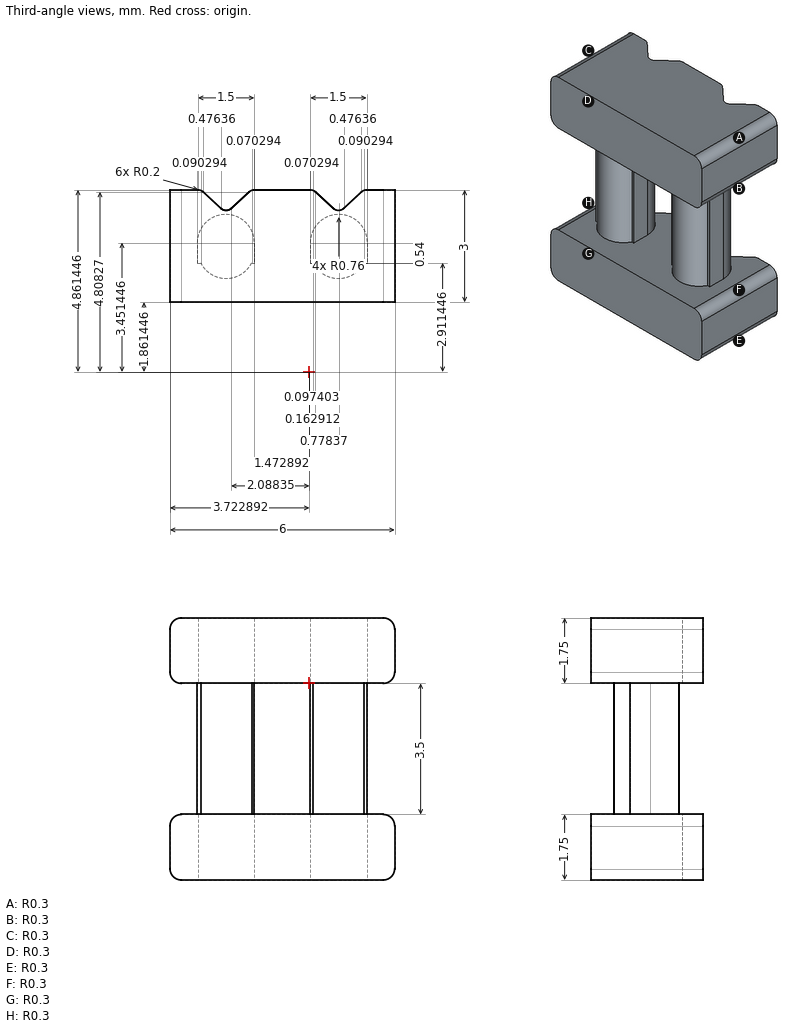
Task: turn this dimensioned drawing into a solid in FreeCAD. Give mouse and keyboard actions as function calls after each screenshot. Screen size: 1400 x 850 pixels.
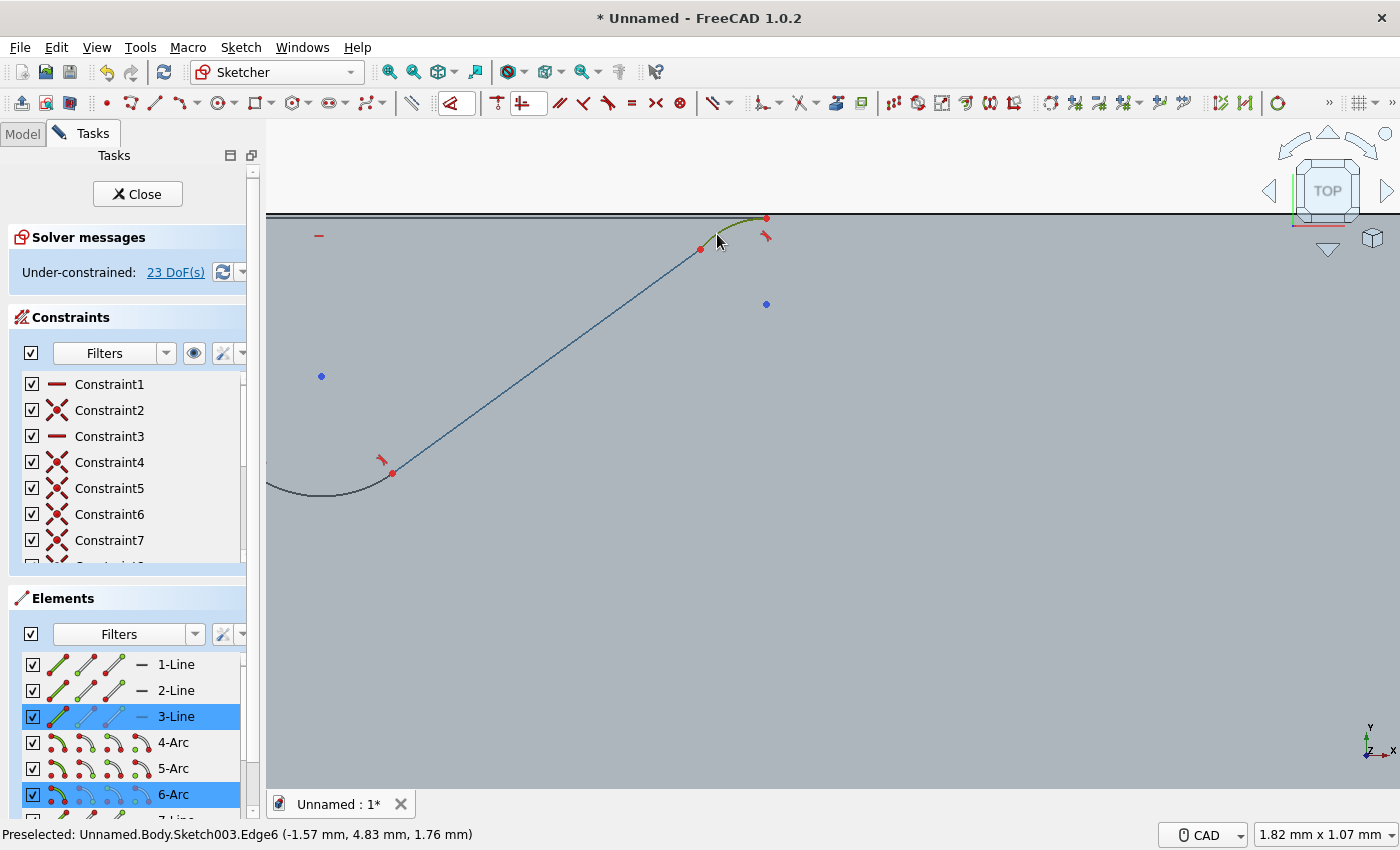
click(608, 104)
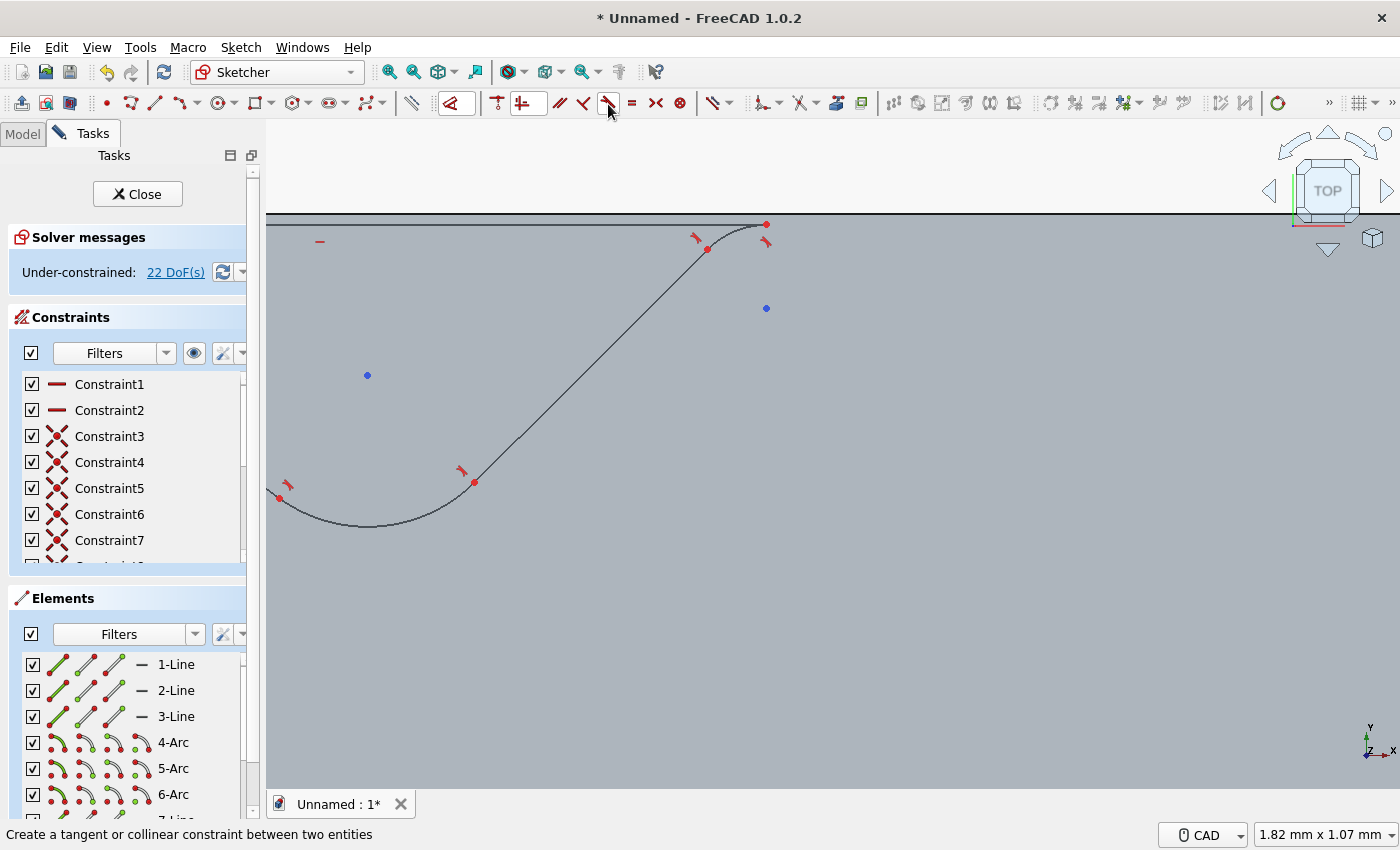
scroll(689, 254, down, 10)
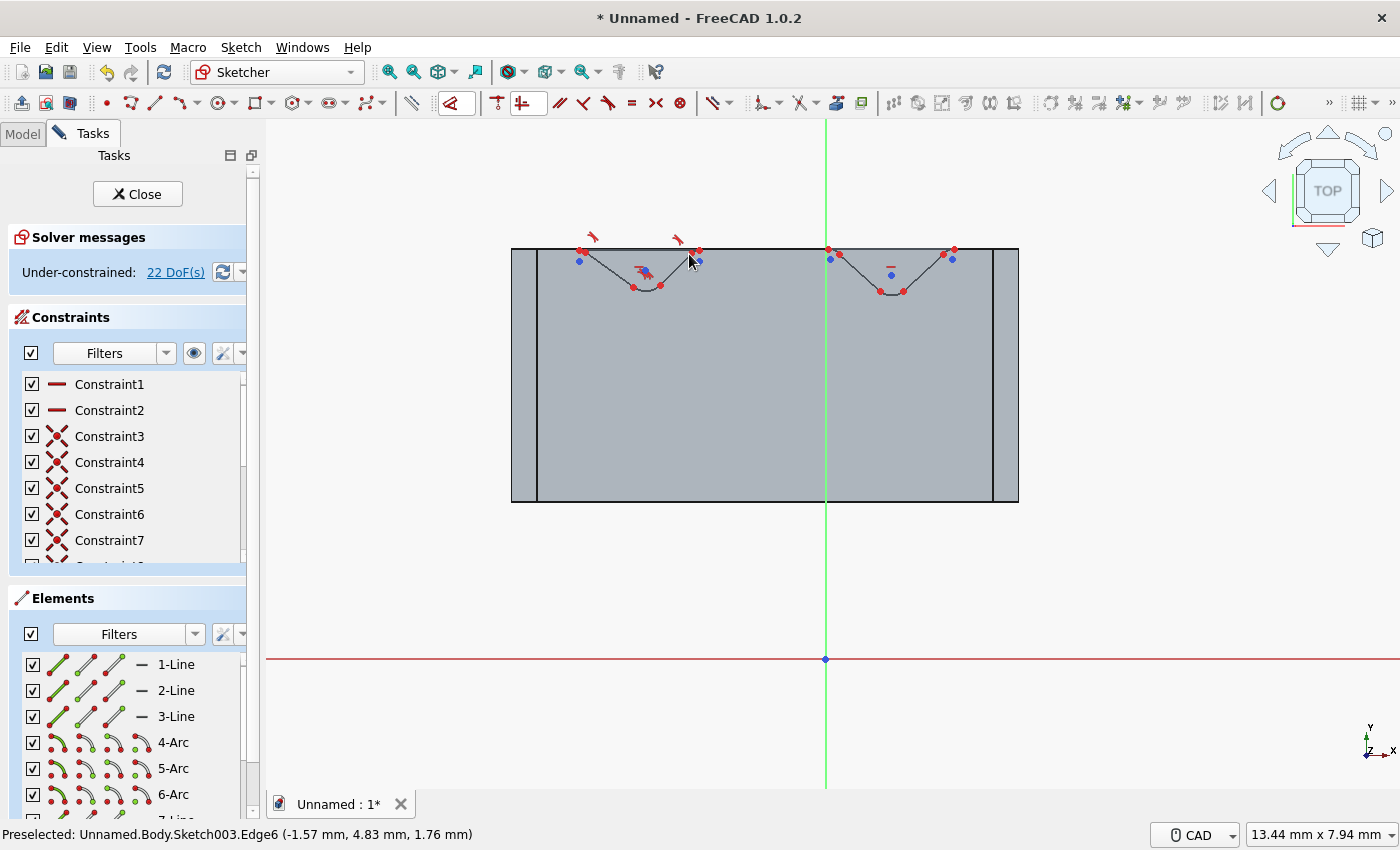
click(852, 266)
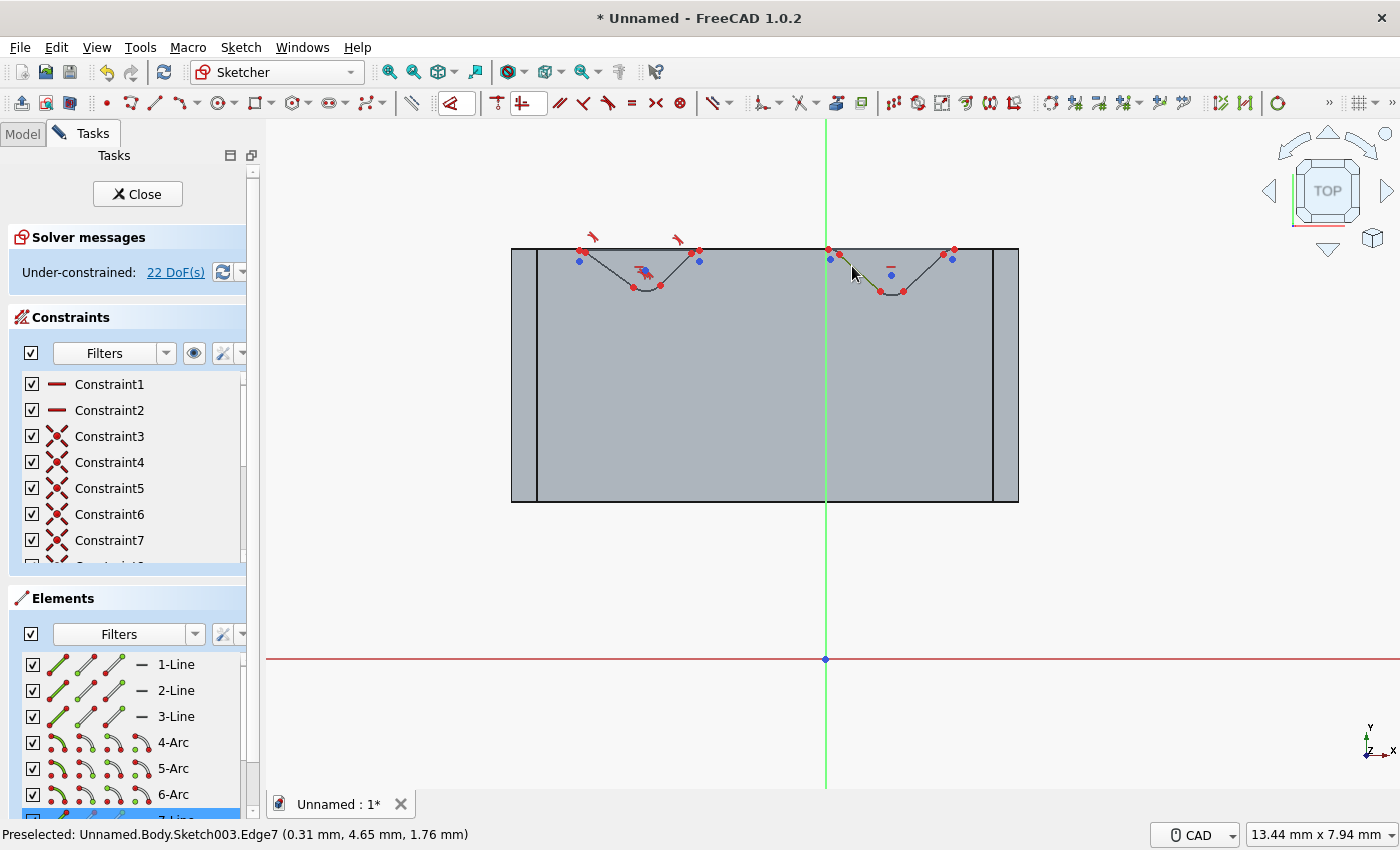
click(892, 295)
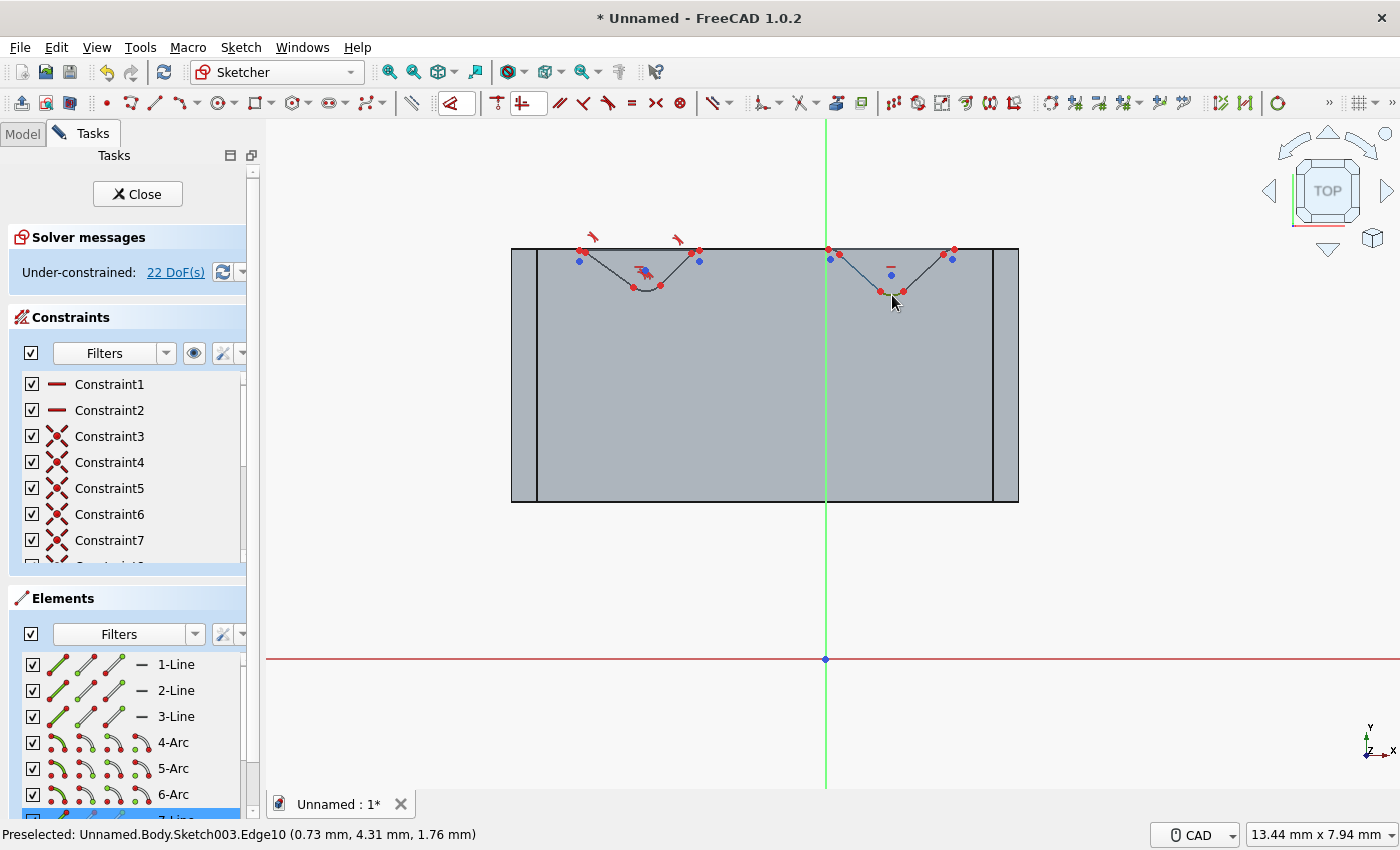
click(608, 104)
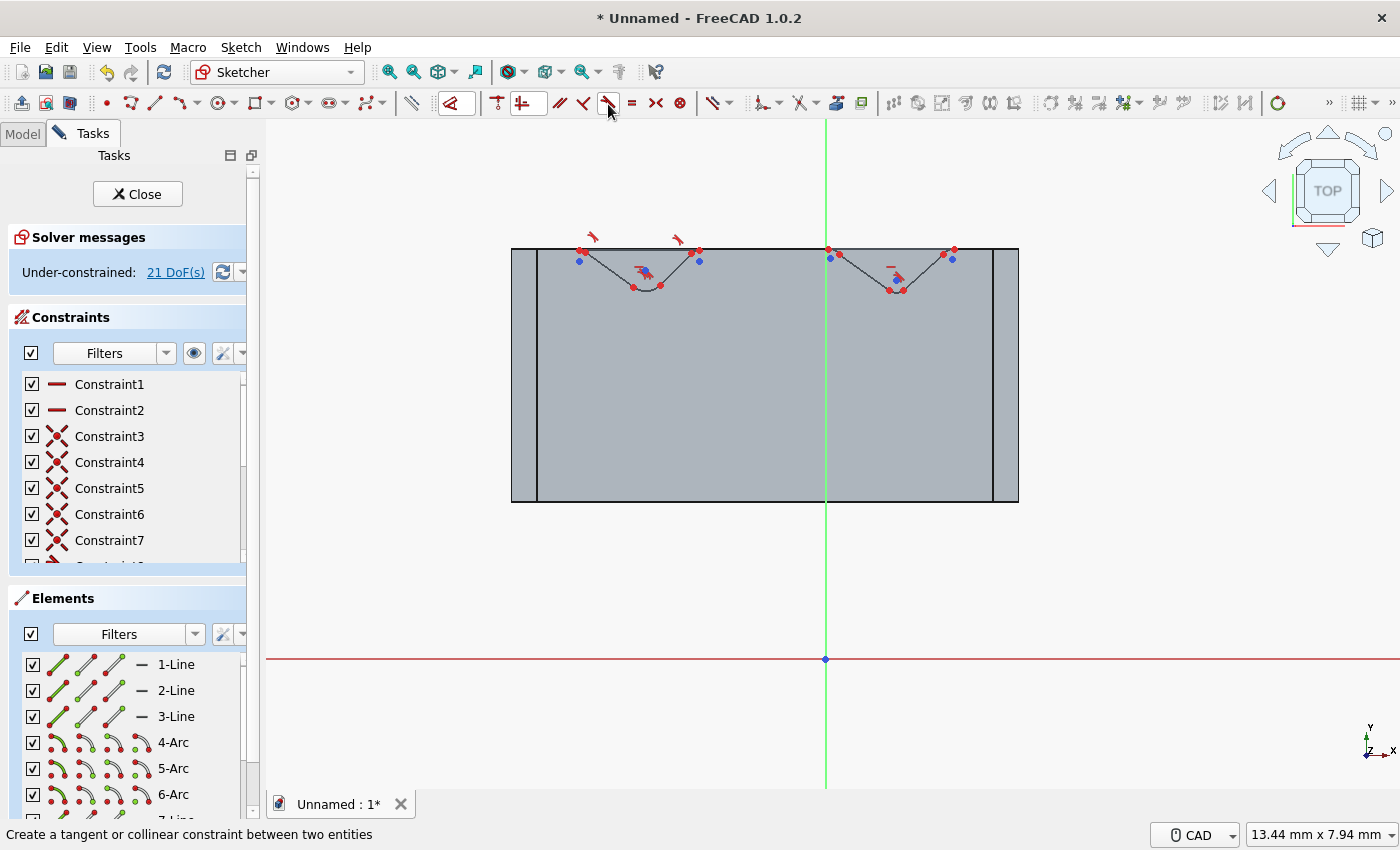
click(854, 265)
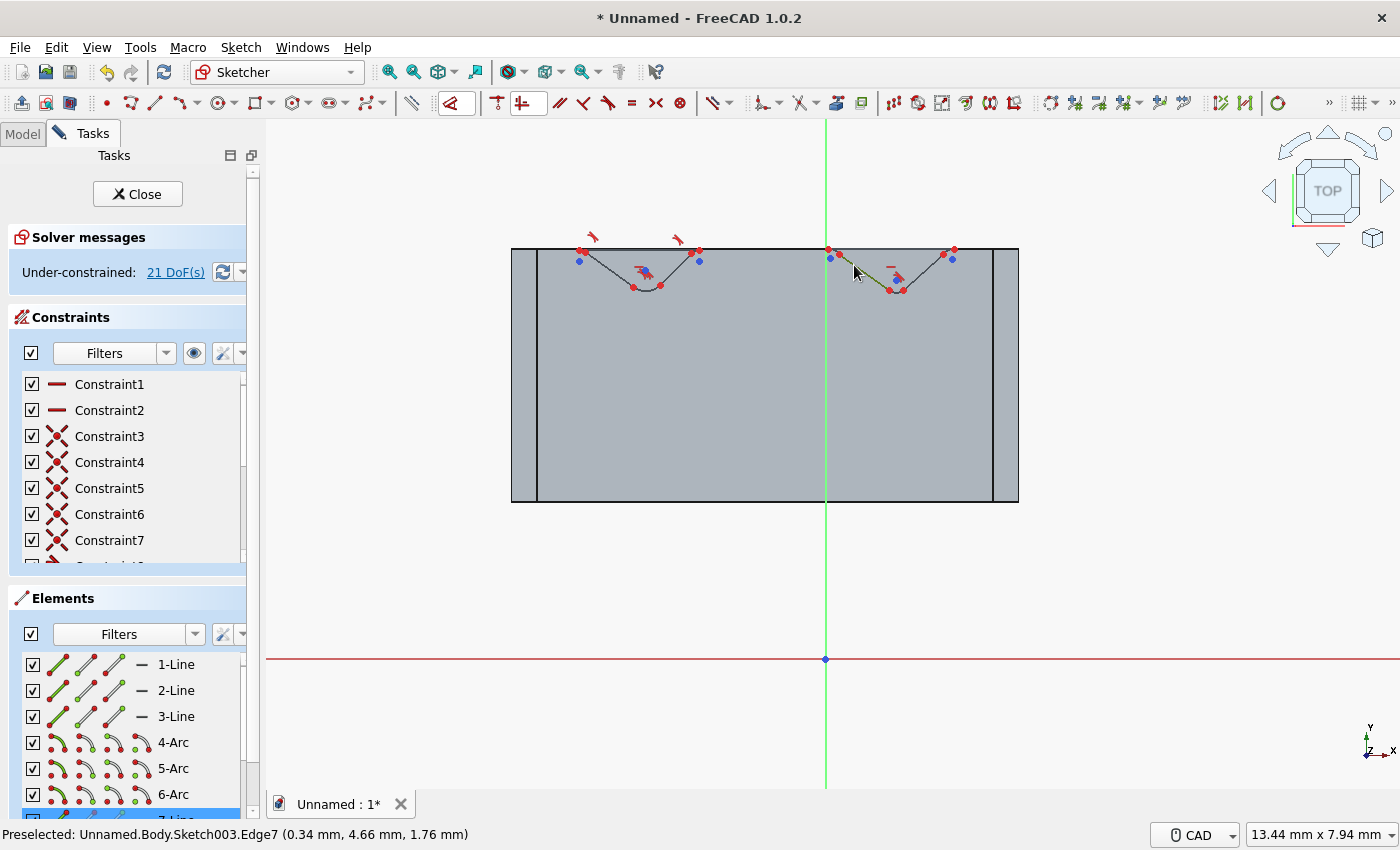
scroll(838, 252, up, 9)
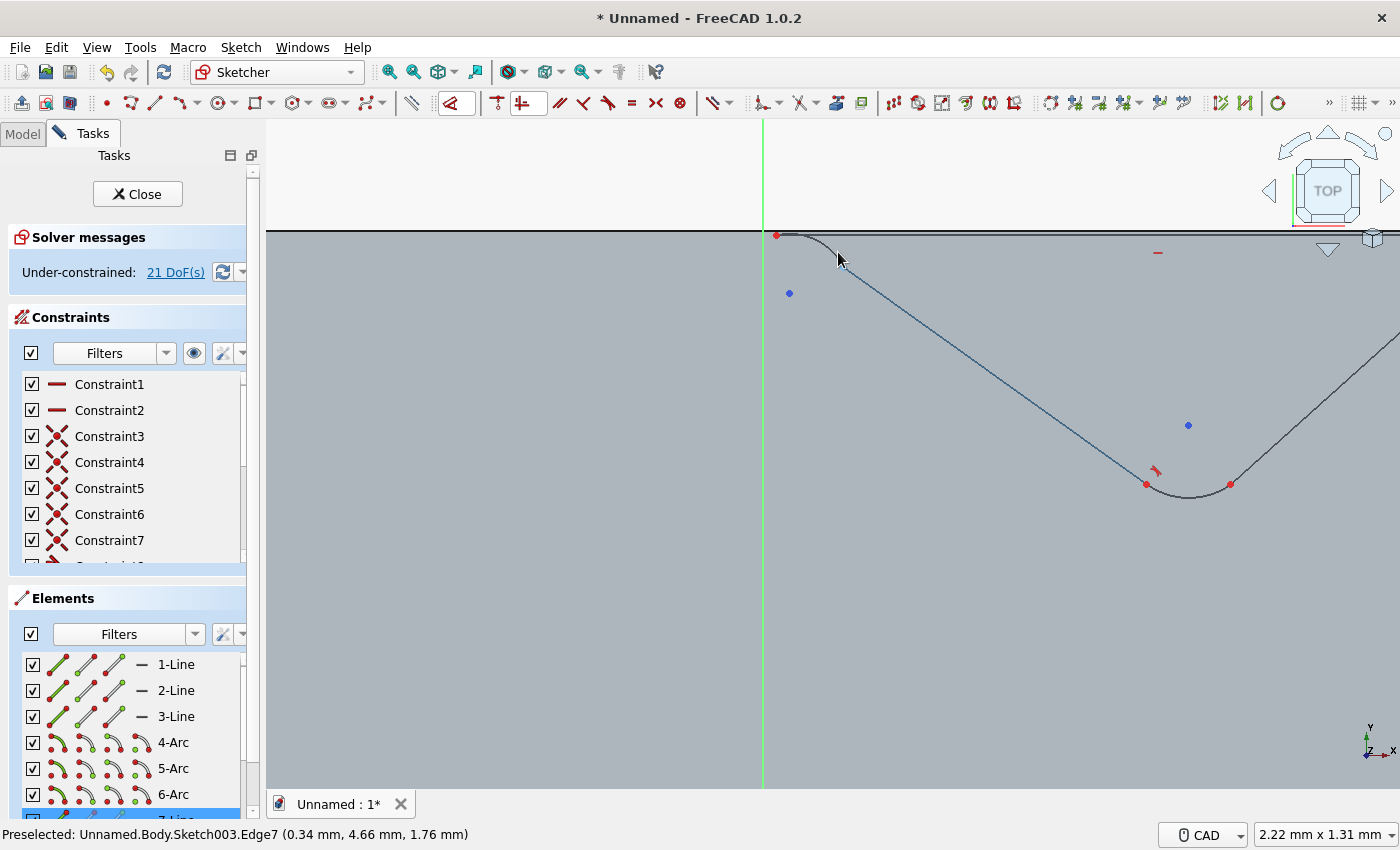
click(834, 254)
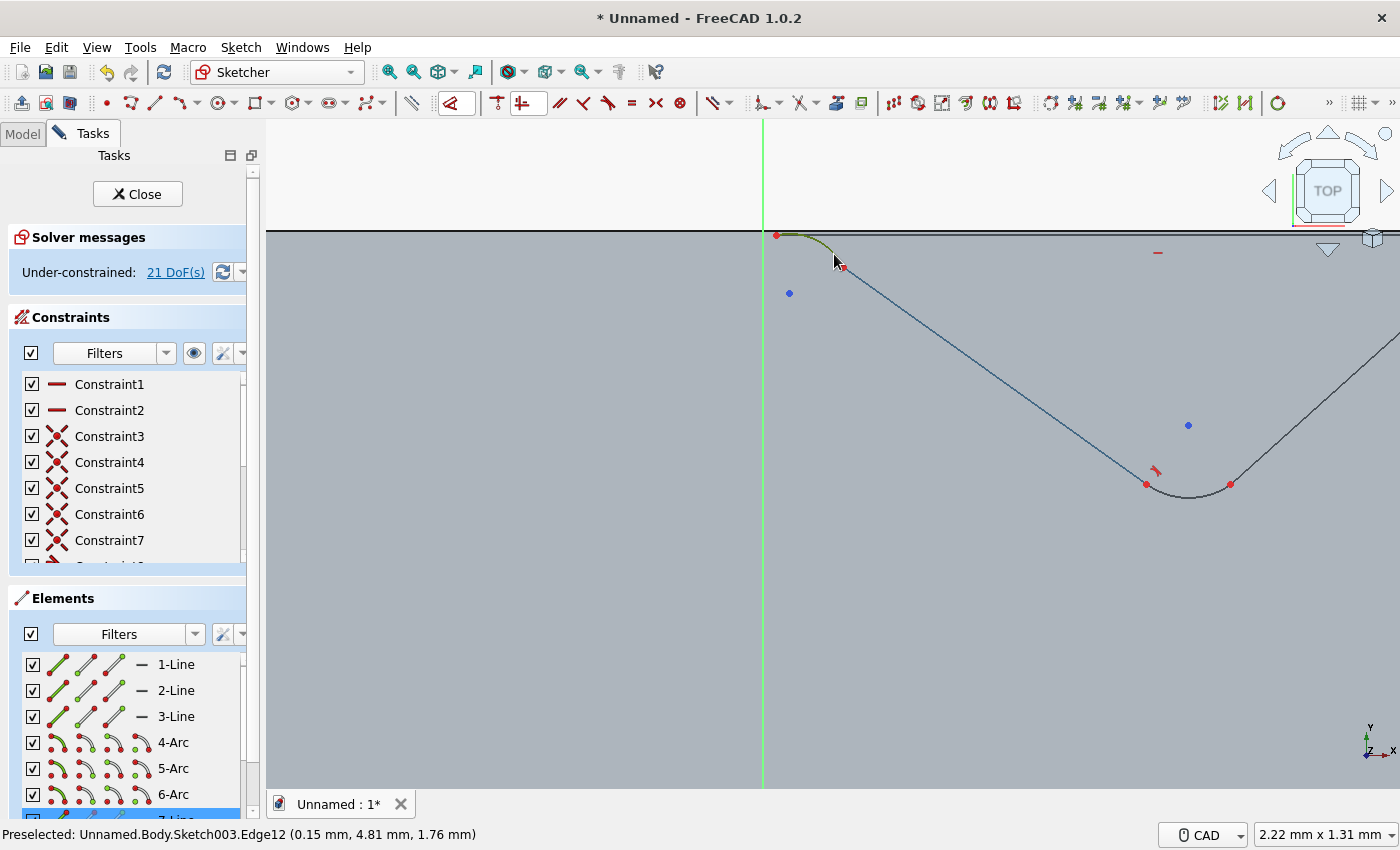
click(608, 104)